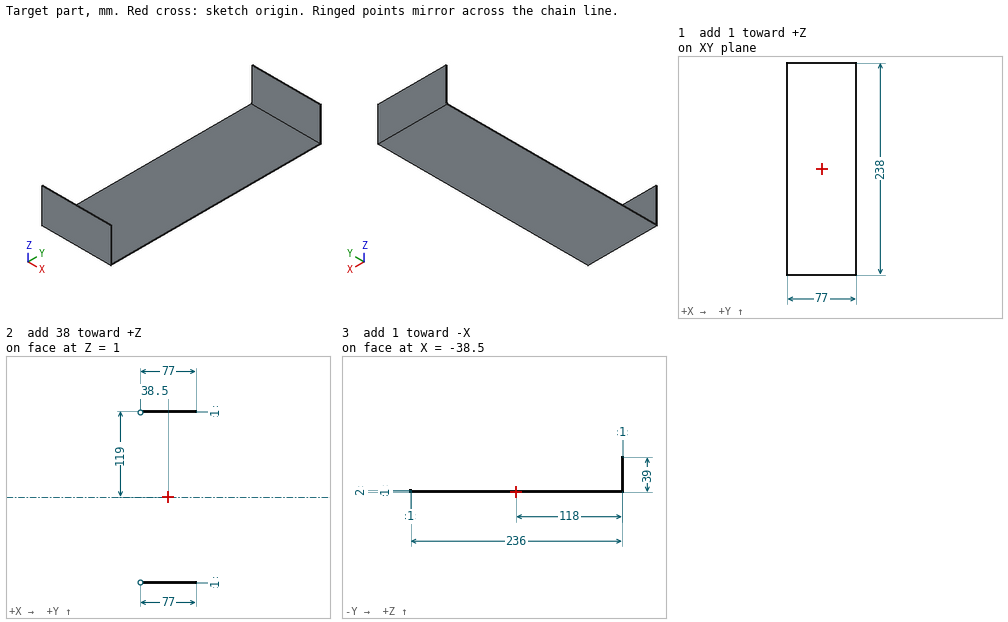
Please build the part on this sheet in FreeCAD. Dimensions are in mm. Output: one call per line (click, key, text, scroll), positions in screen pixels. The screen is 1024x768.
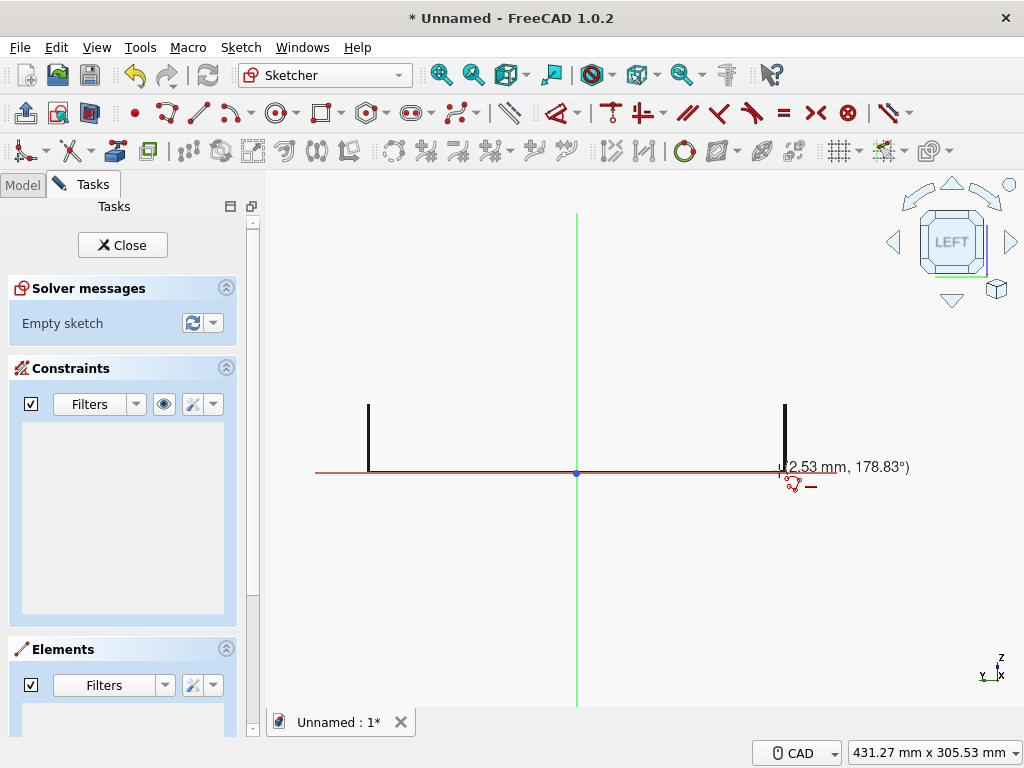
scroll(369, 472, up, 12)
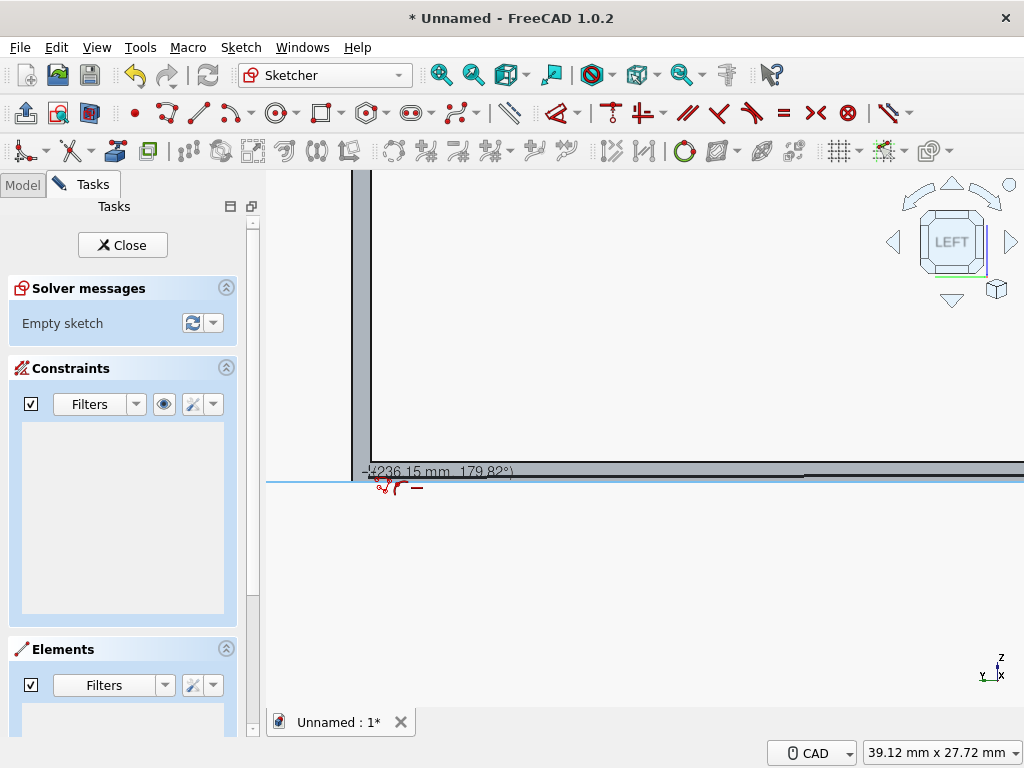
click(371, 462)
click(371, 443)
click(352, 443)
click(352, 482)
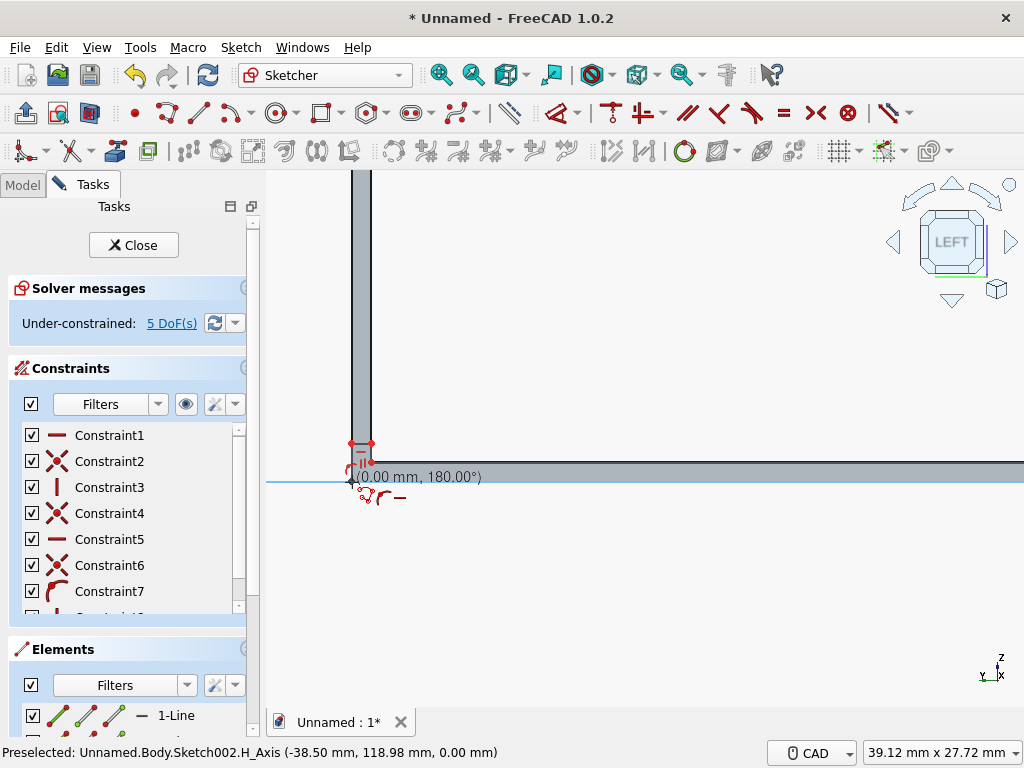
scroll(369, 472, down, 12)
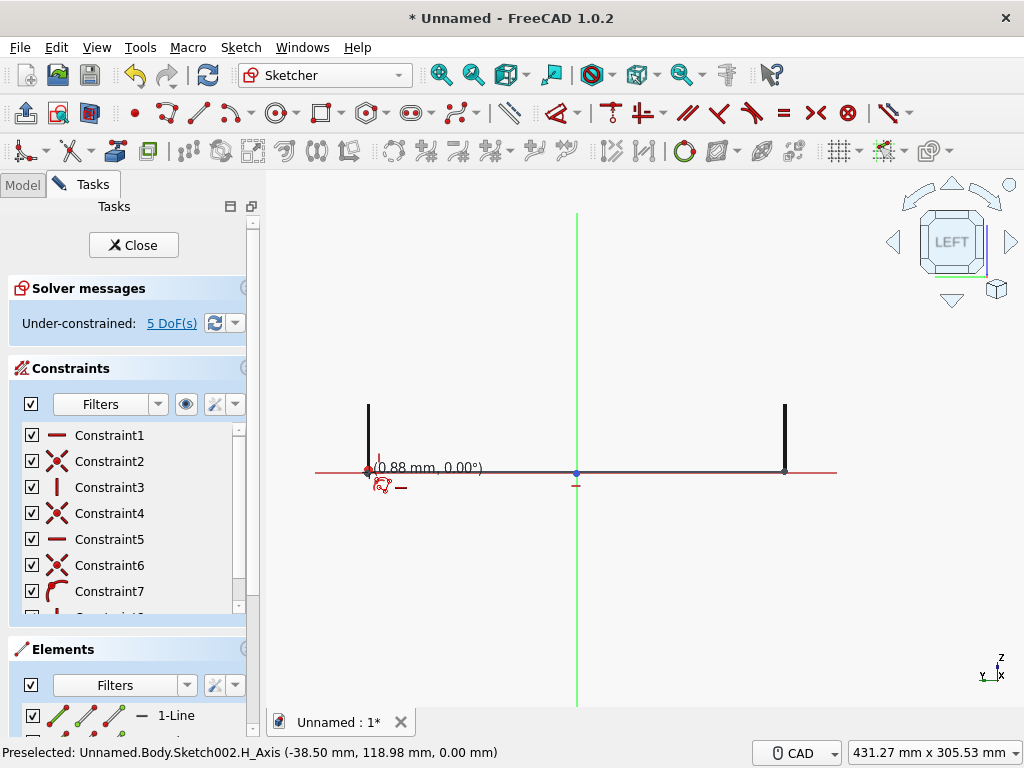
scroll(786, 473, up, 10)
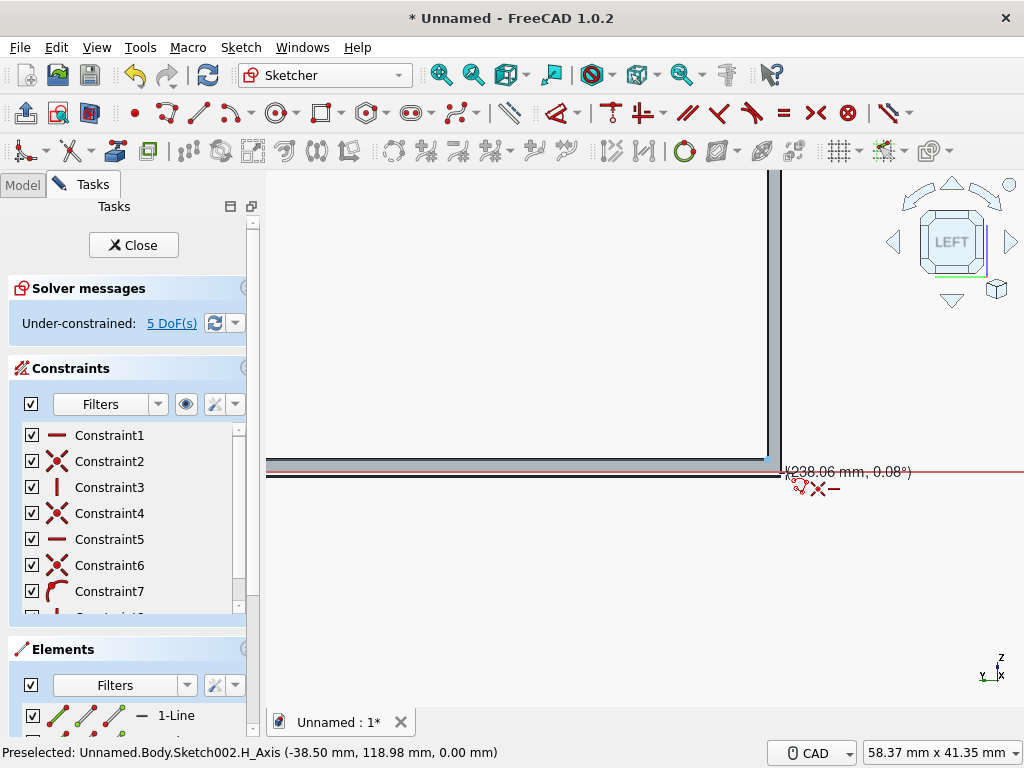
click(781, 463)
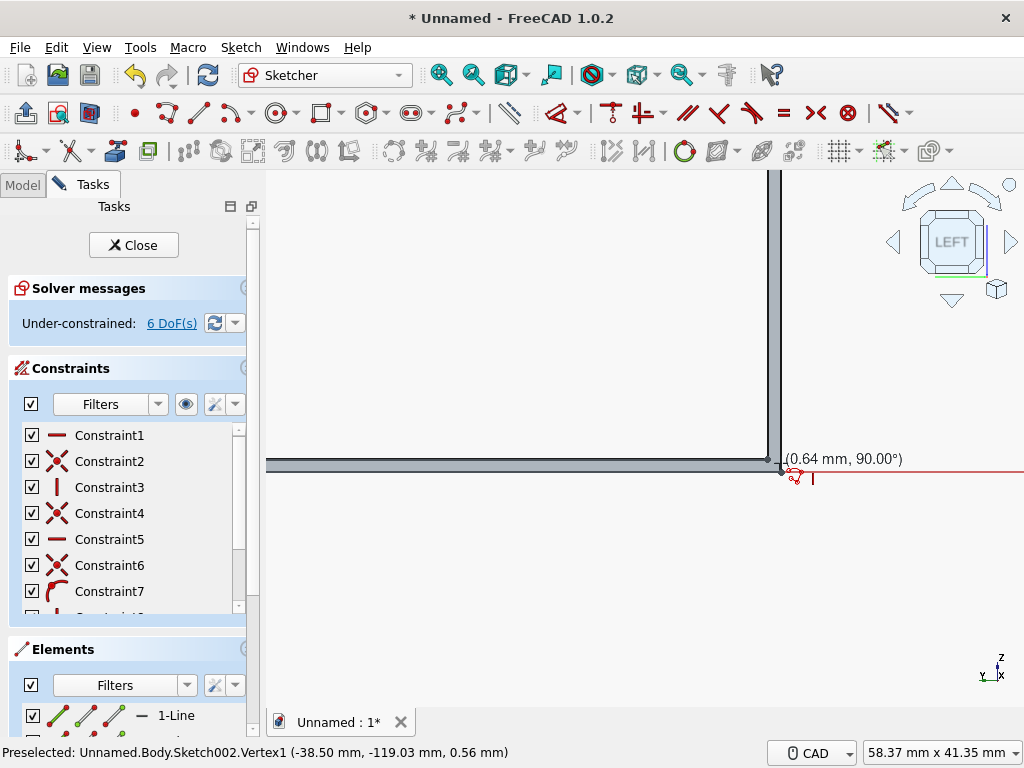
scroll(786, 473, down, 10)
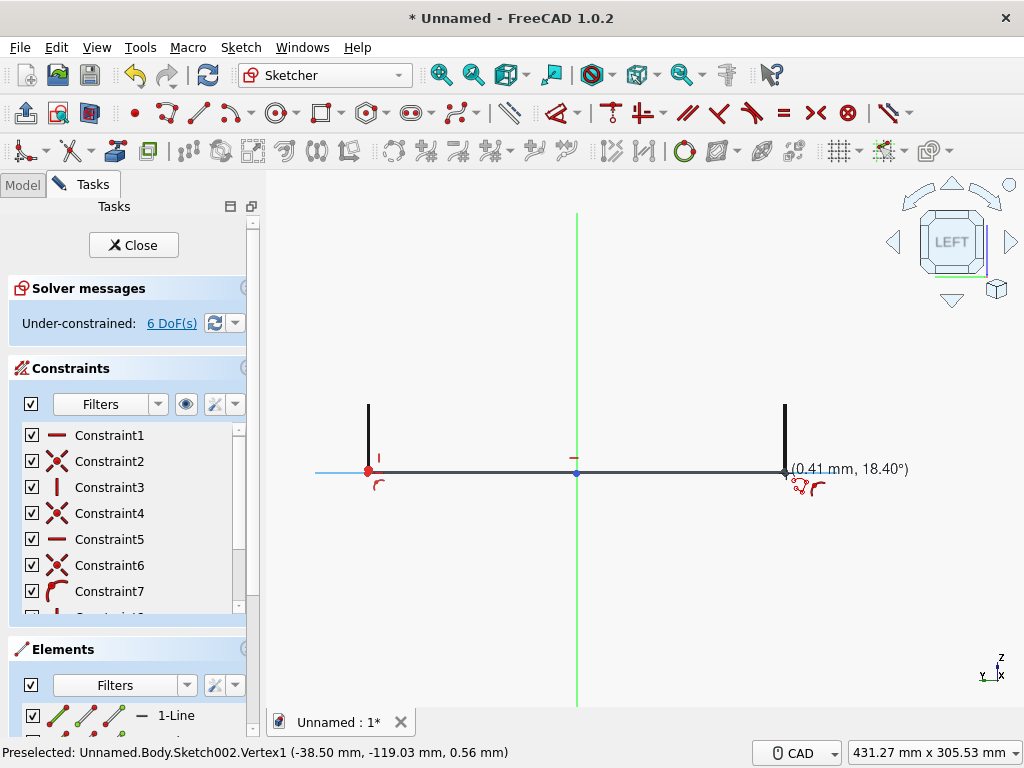
click(786, 405)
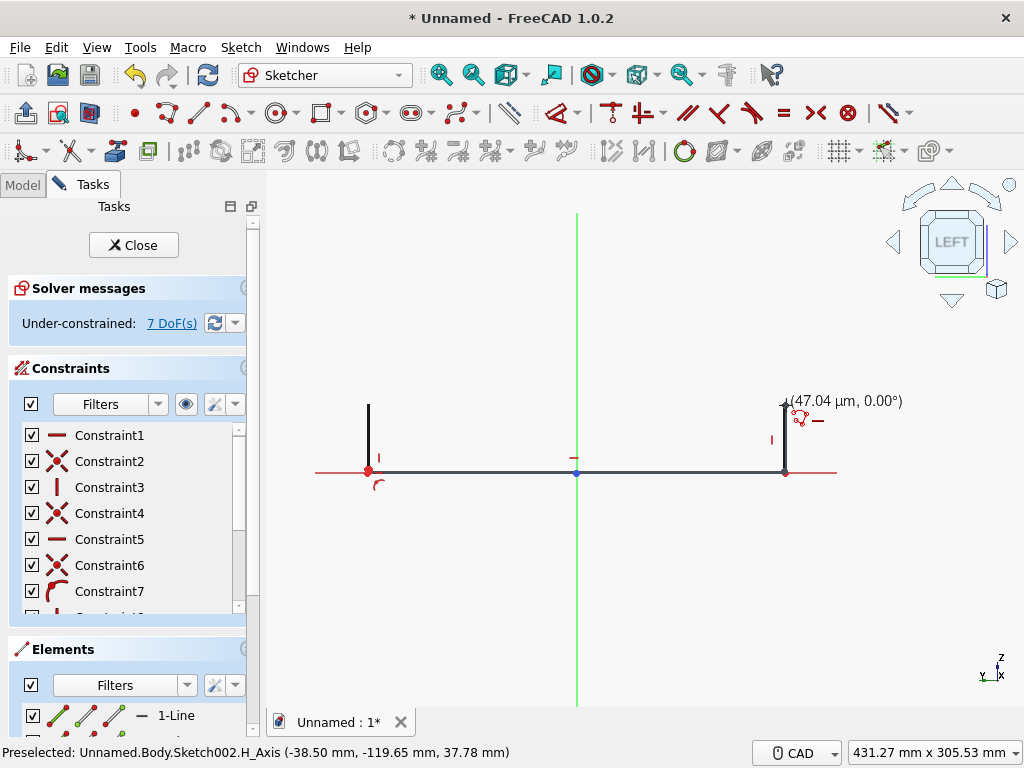
scroll(784, 405, up, 12)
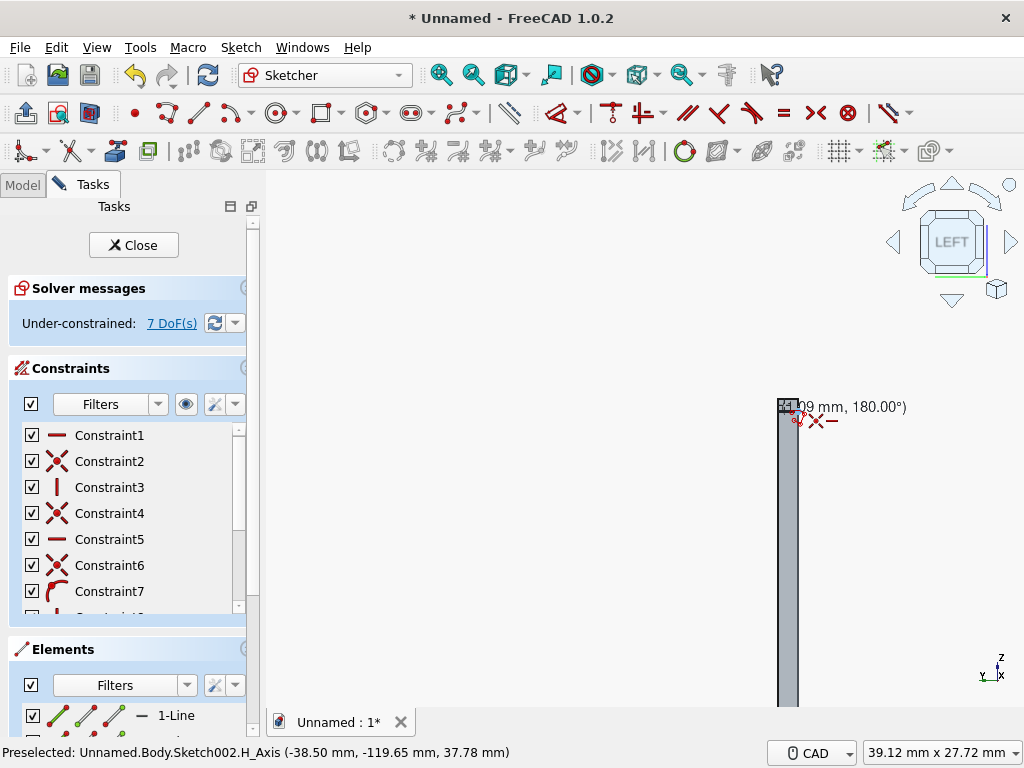
click(778, 401)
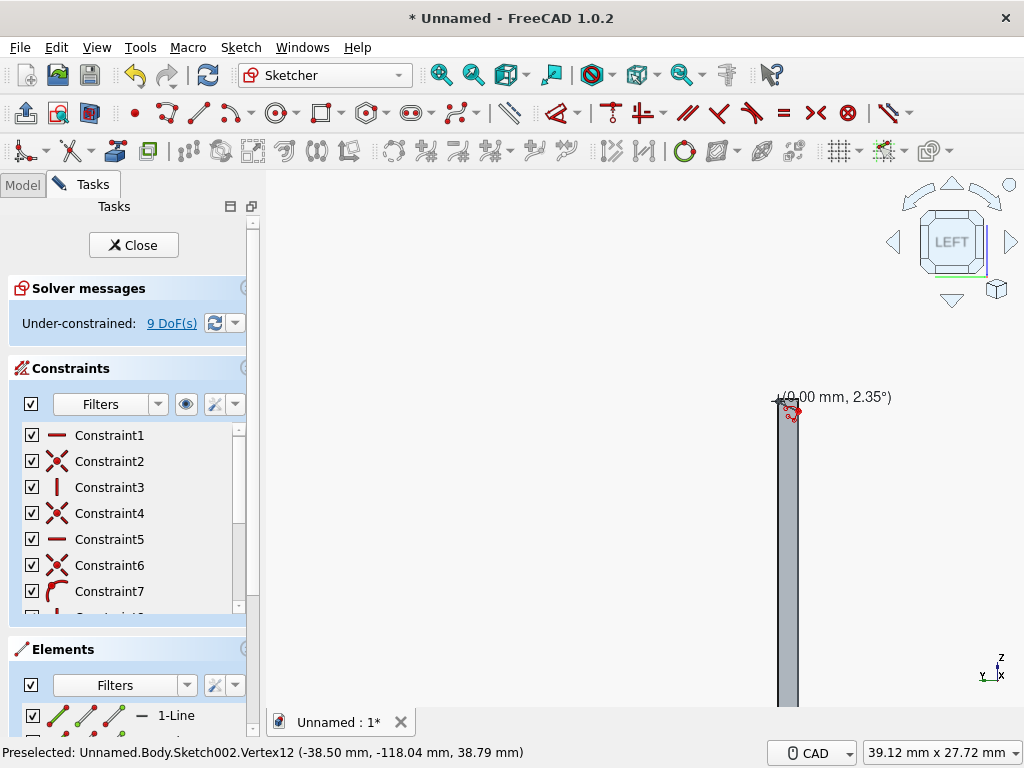
scroll(784, 405, down, 12)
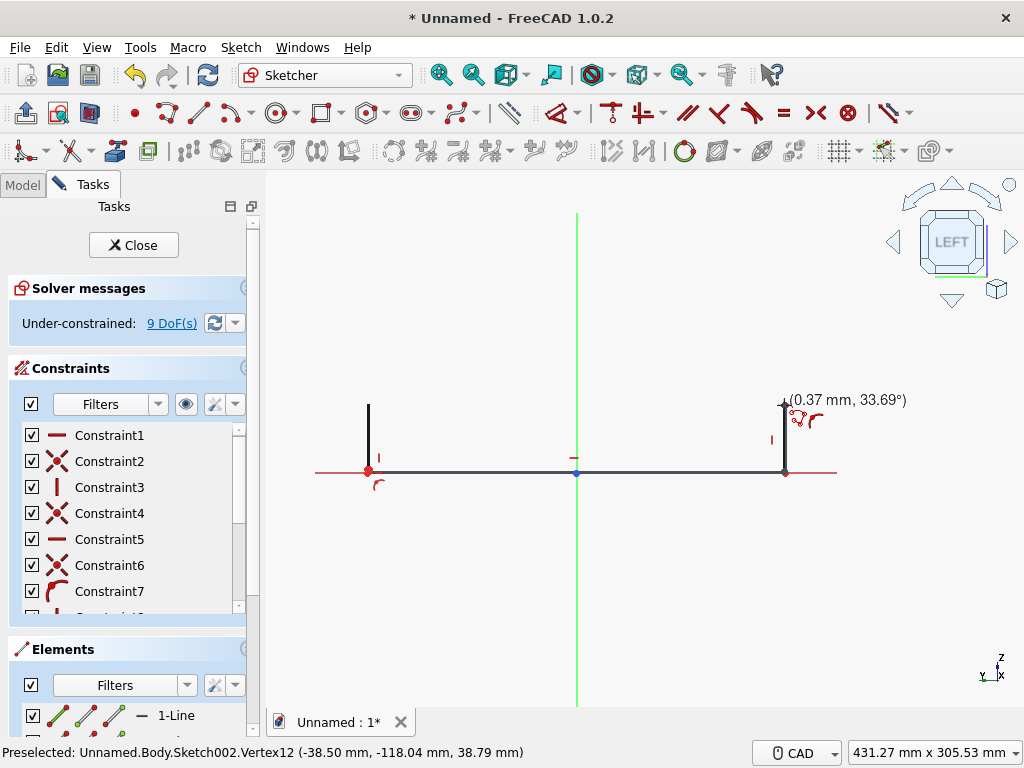
scroll(784, 472, up, 12)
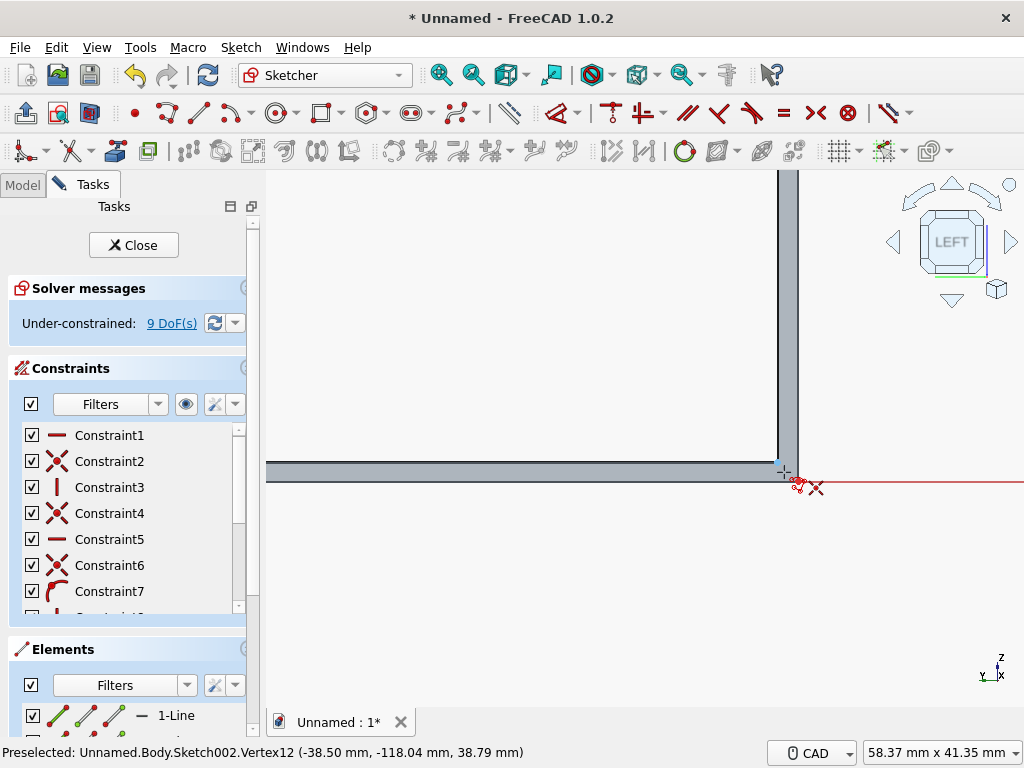
click(778, 463)
key(Escape)
key(Escape)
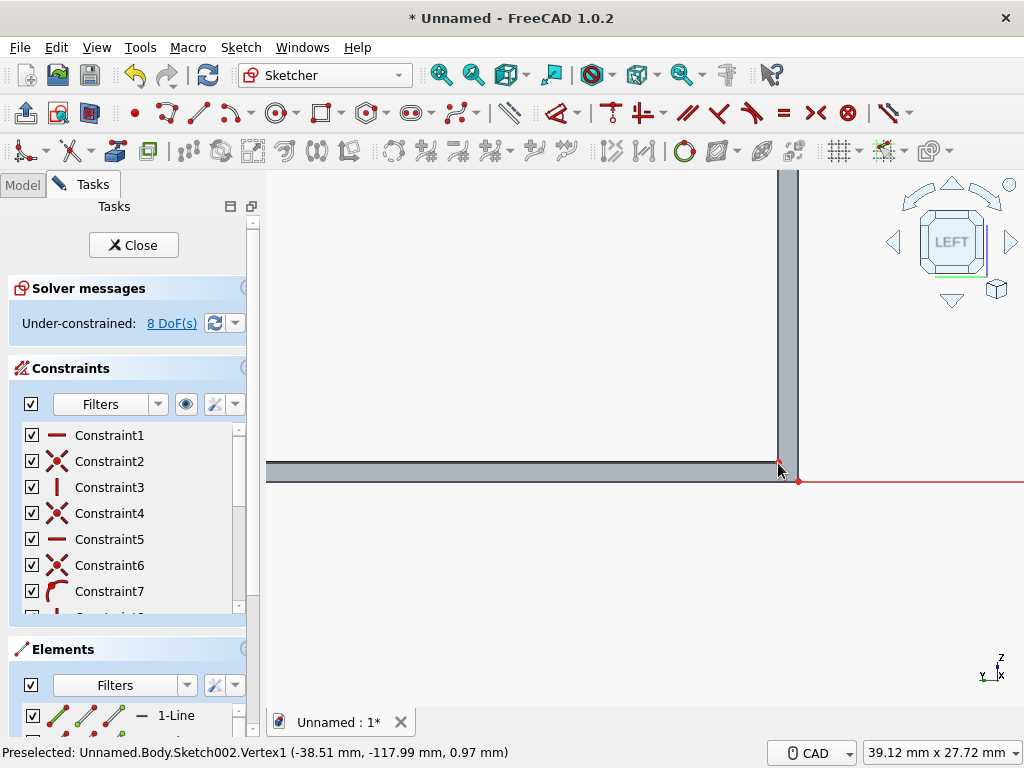
scroll(784, 472, down, 12)